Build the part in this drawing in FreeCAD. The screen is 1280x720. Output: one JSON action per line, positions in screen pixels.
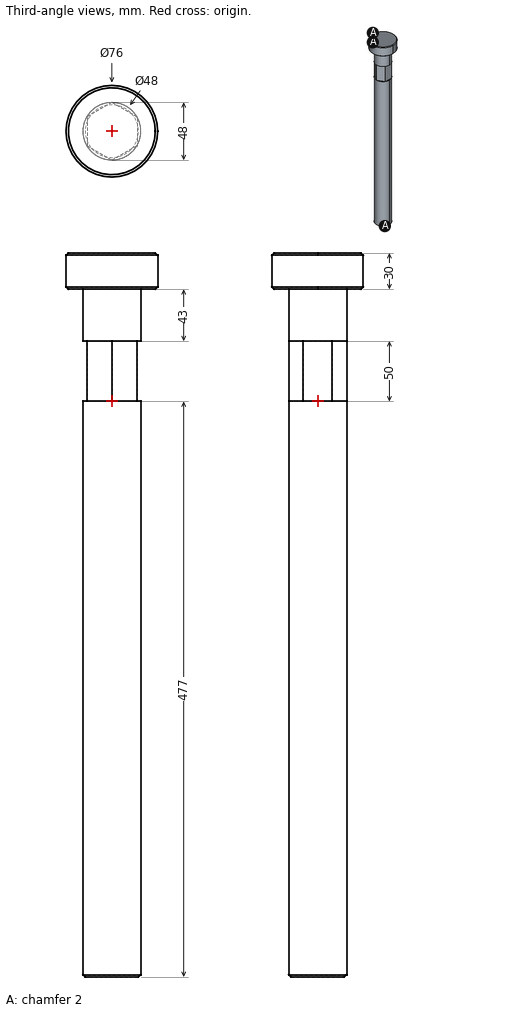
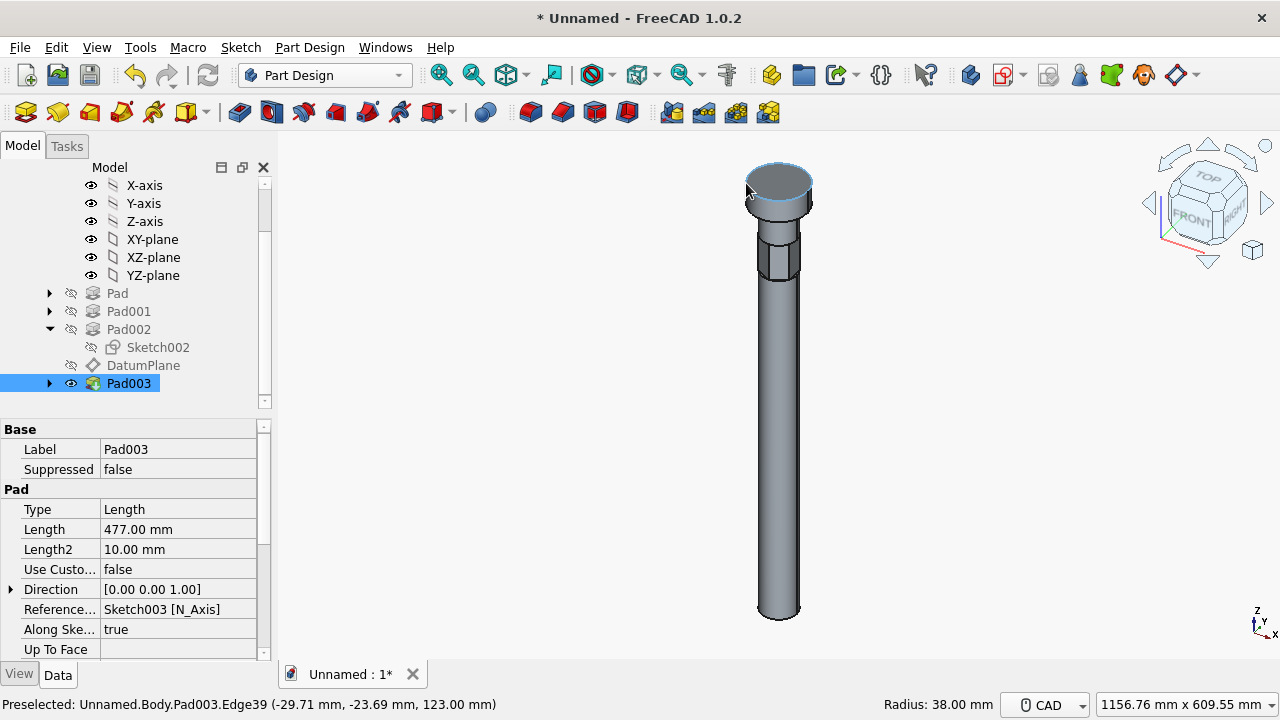
{"action": "left_click", "coordinate": [764, 615], "text": "ctrl"}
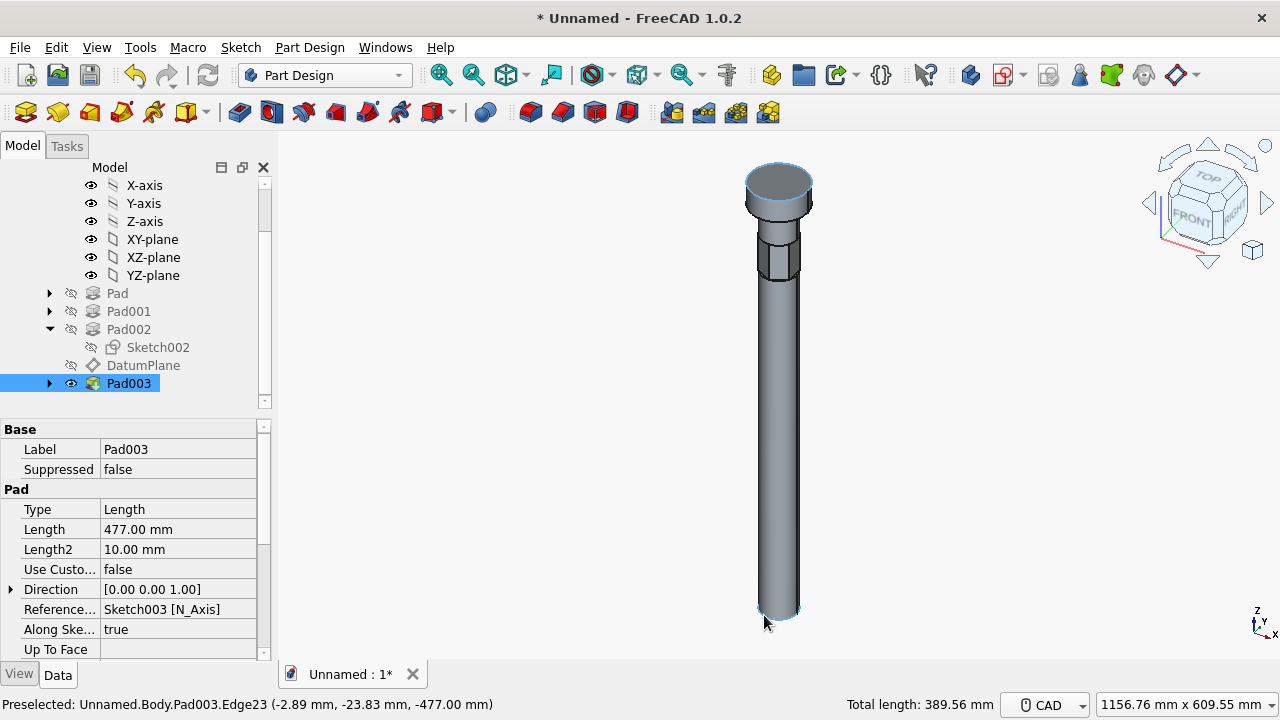
{"action": "key", "text": "0"}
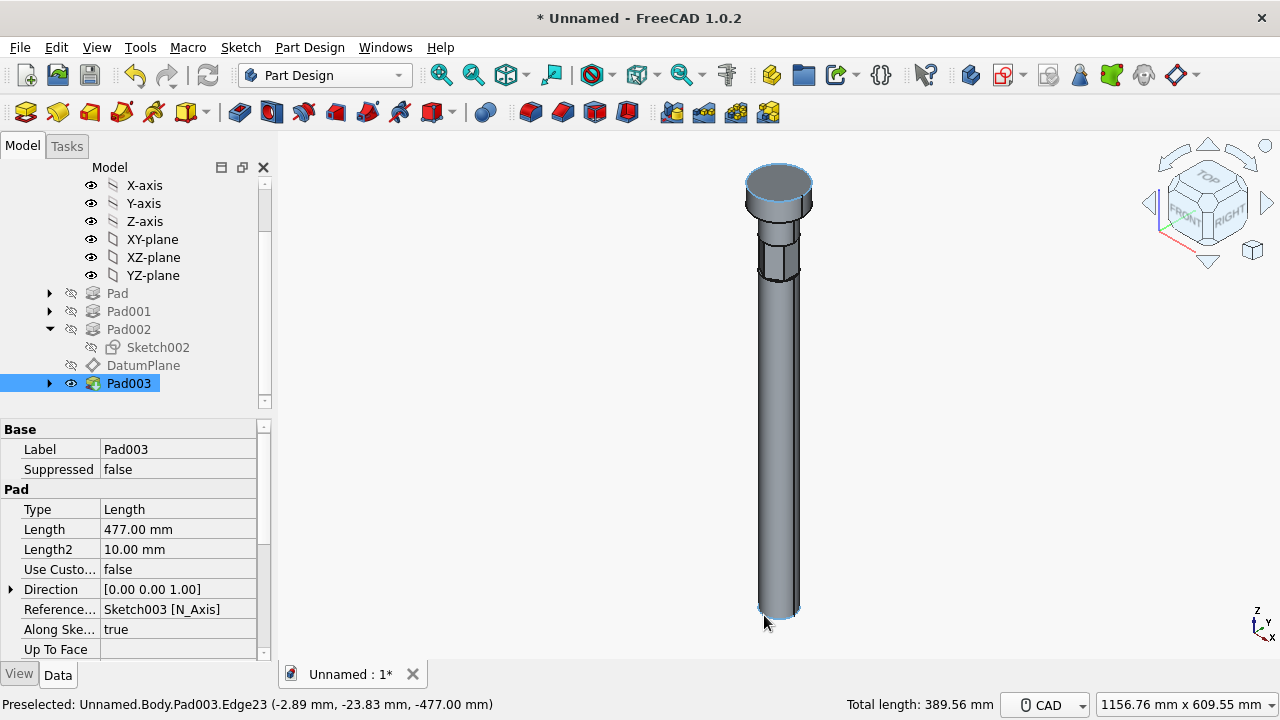
{"action": "key", "text": "2"}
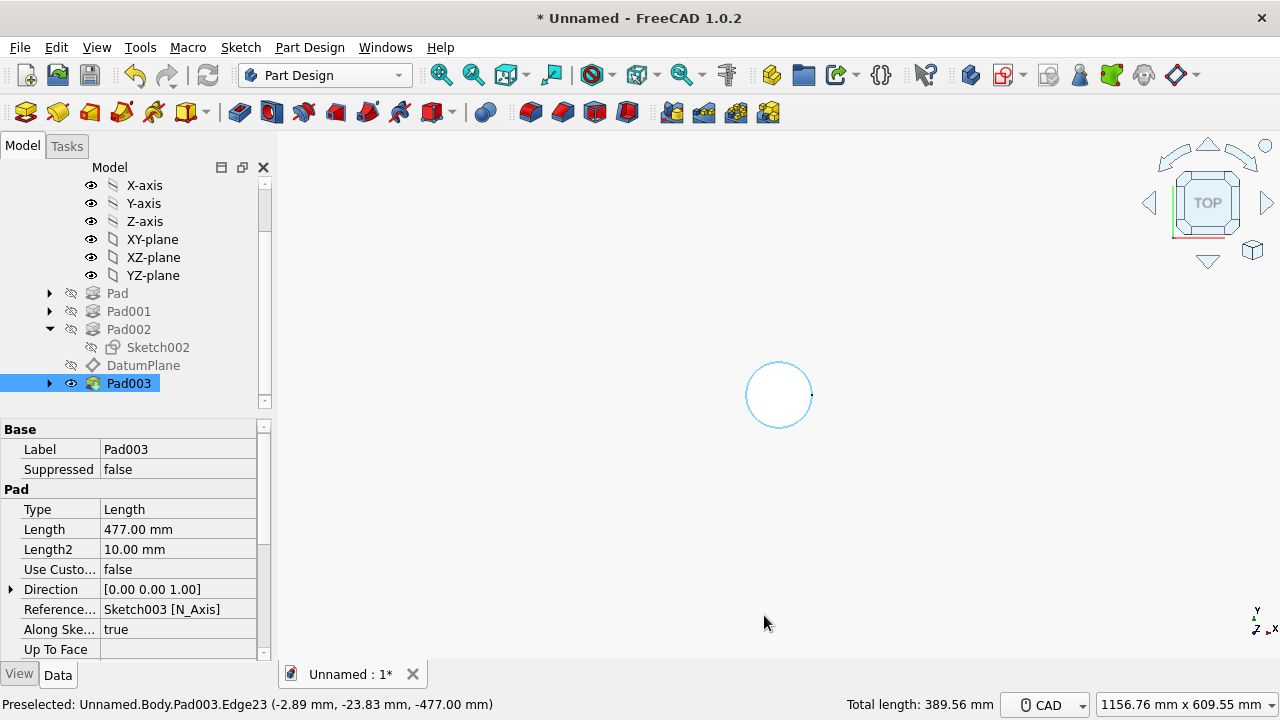
{"action": "left_click", "coordinate": [442, 76]}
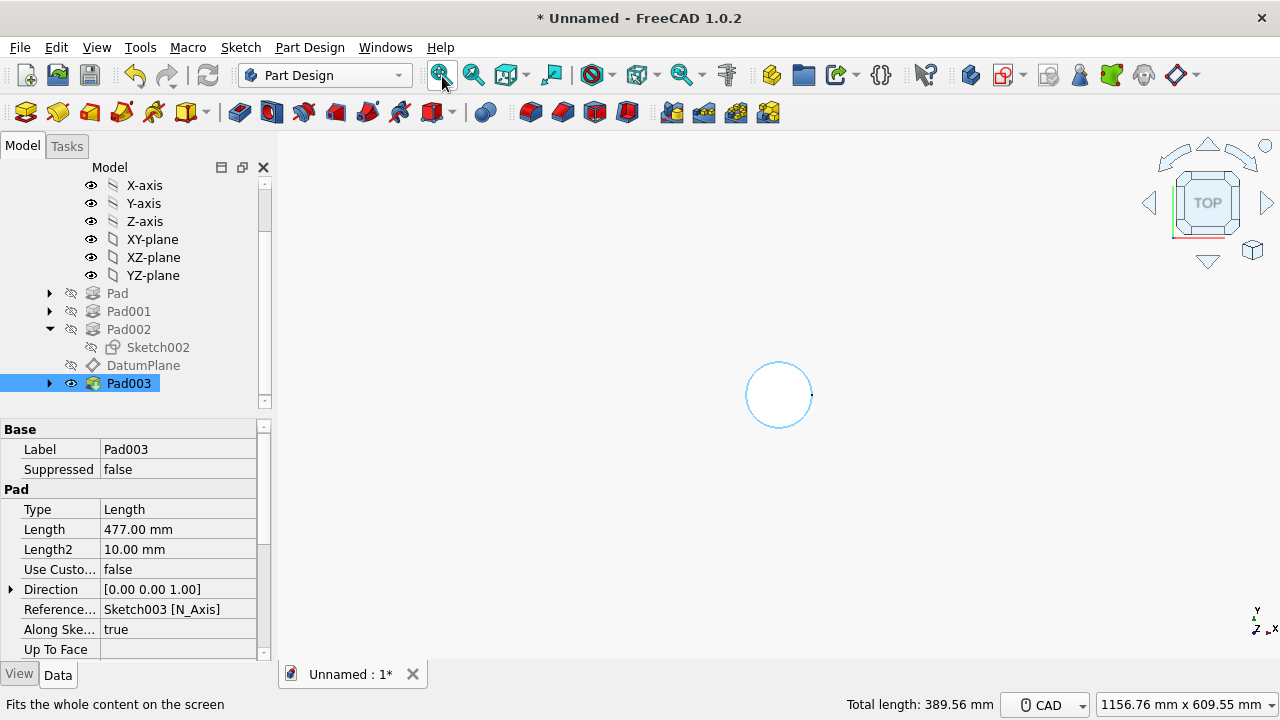
{"action": "key", "text": "1"}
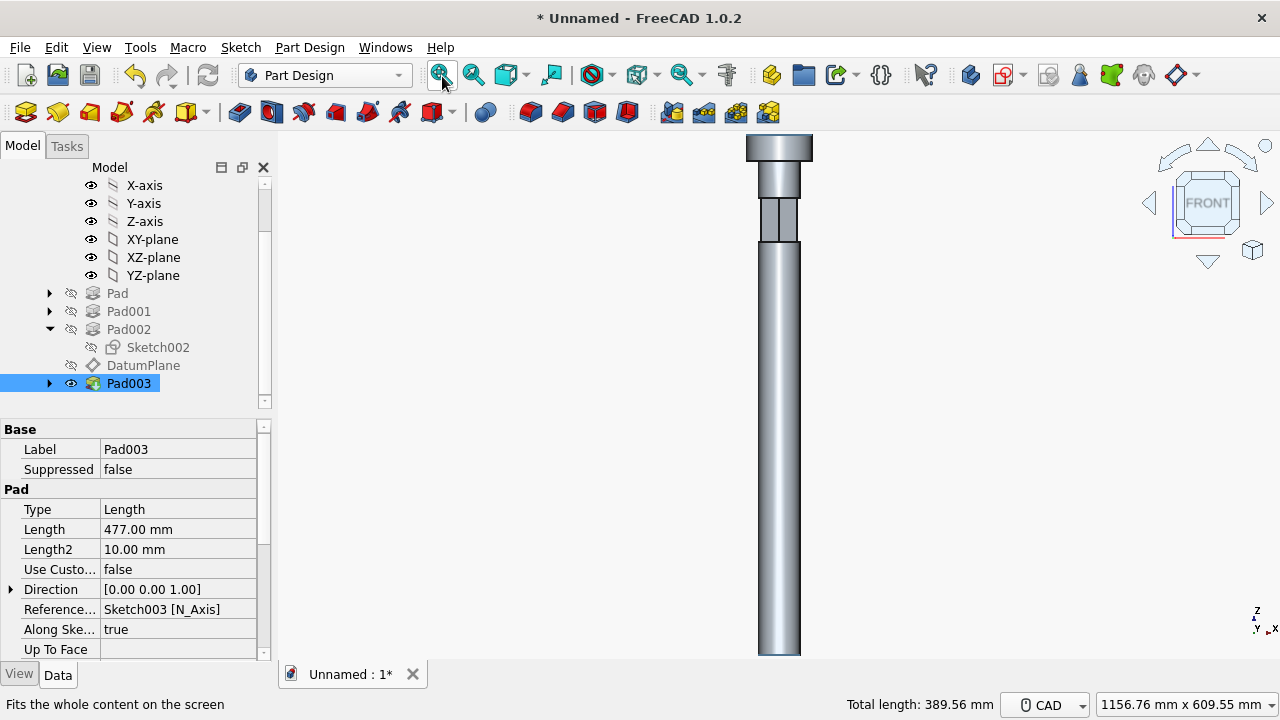
{"action": "left_click", "coordinate": [752, 160], "text": "ctrl"}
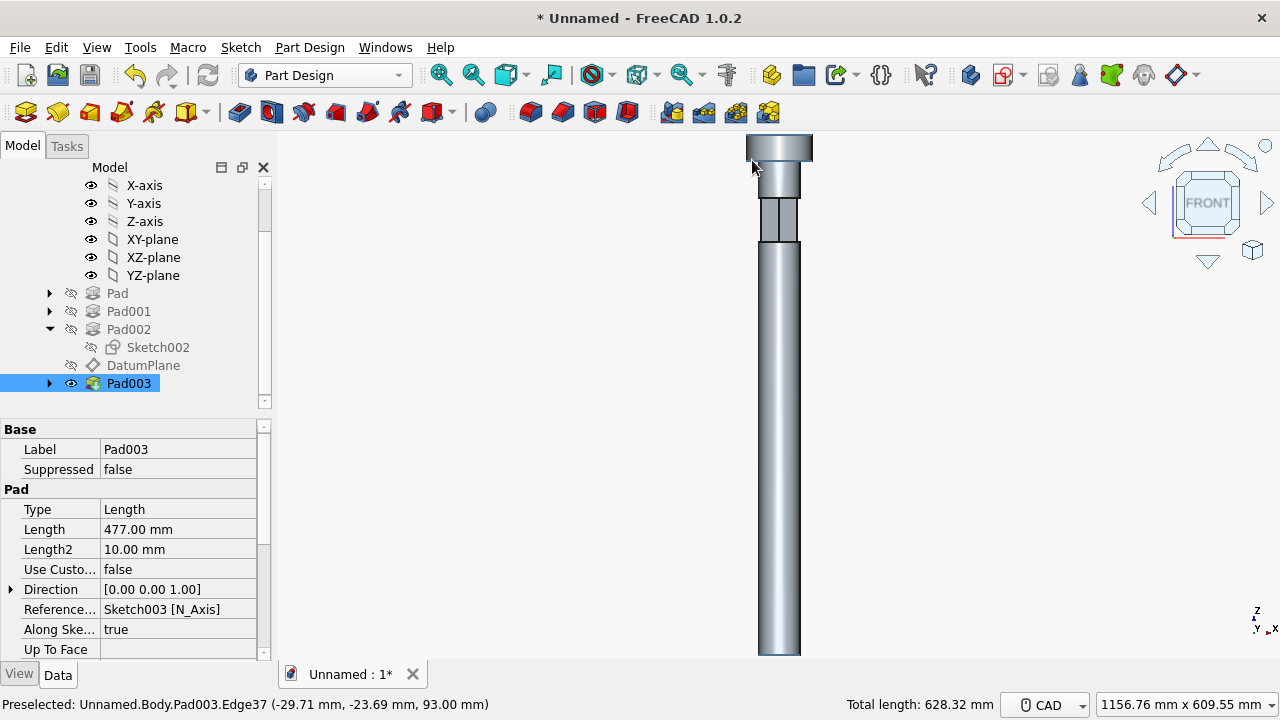
{"action": "left_click", "coordinate": [564, 112]}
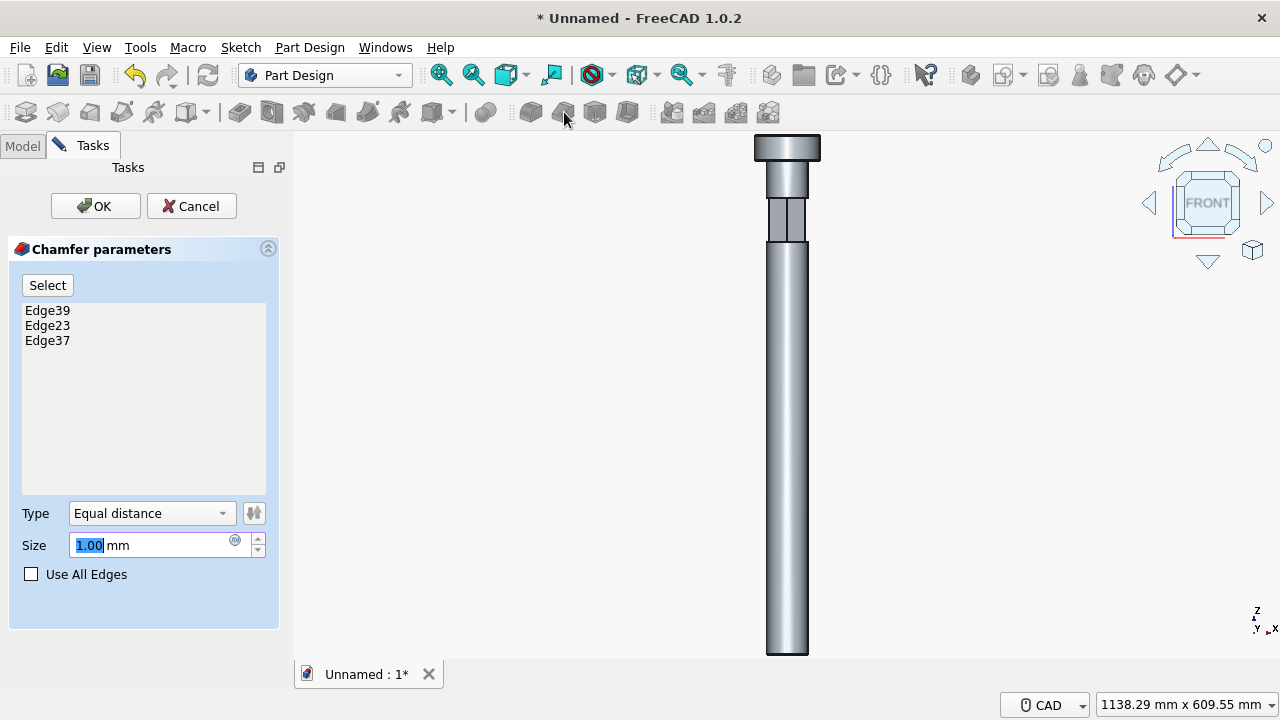
{"action": "type", "text": "2"}
{"action": "key", "text": "Tab"}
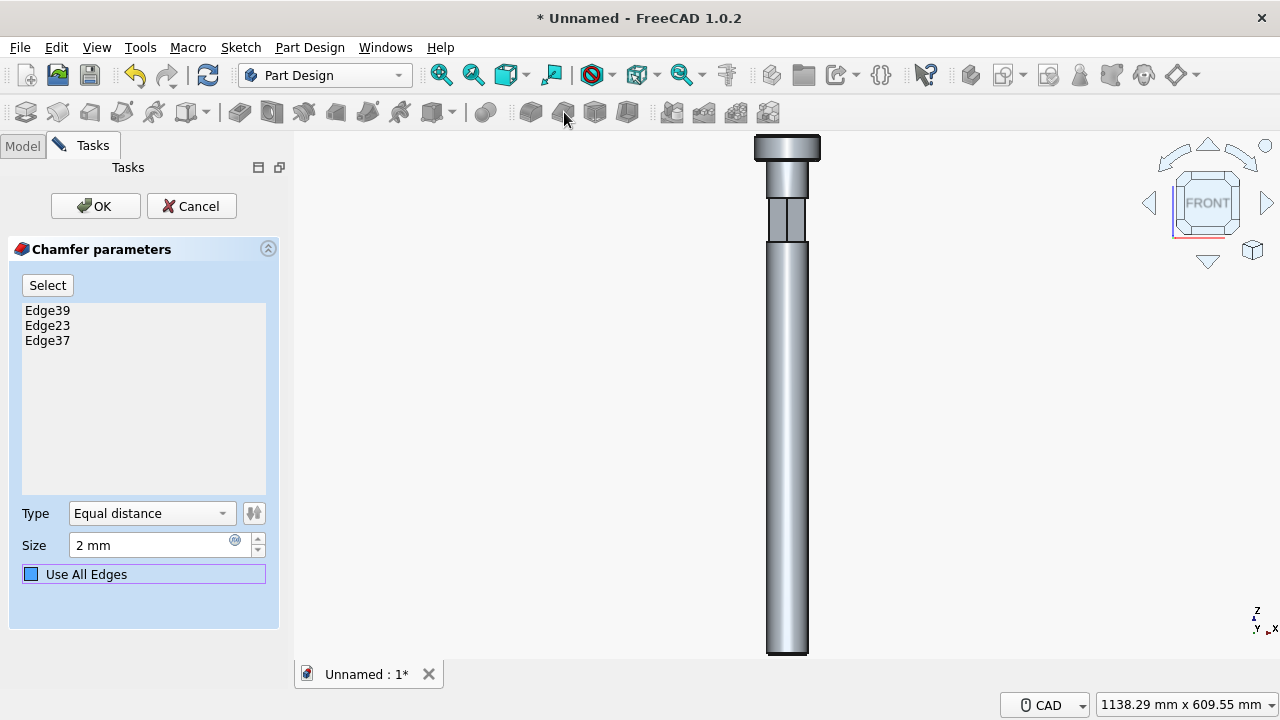
{"action": "left_click", "coordinate": [96, 206]}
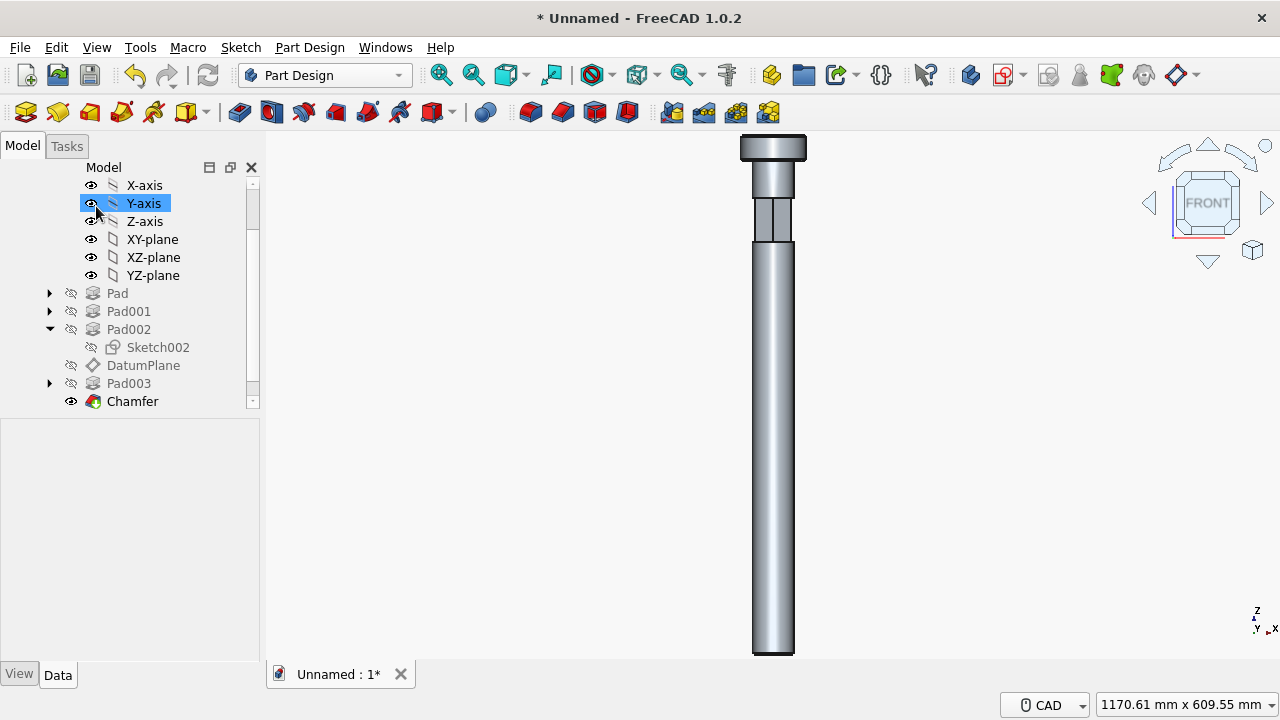
{"action": "key", "text": "0"}